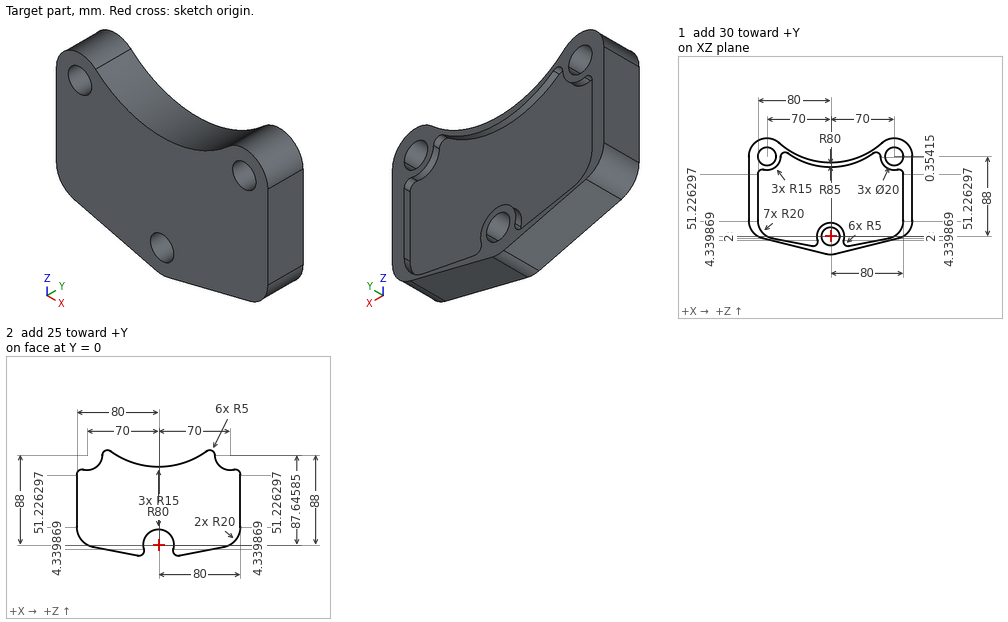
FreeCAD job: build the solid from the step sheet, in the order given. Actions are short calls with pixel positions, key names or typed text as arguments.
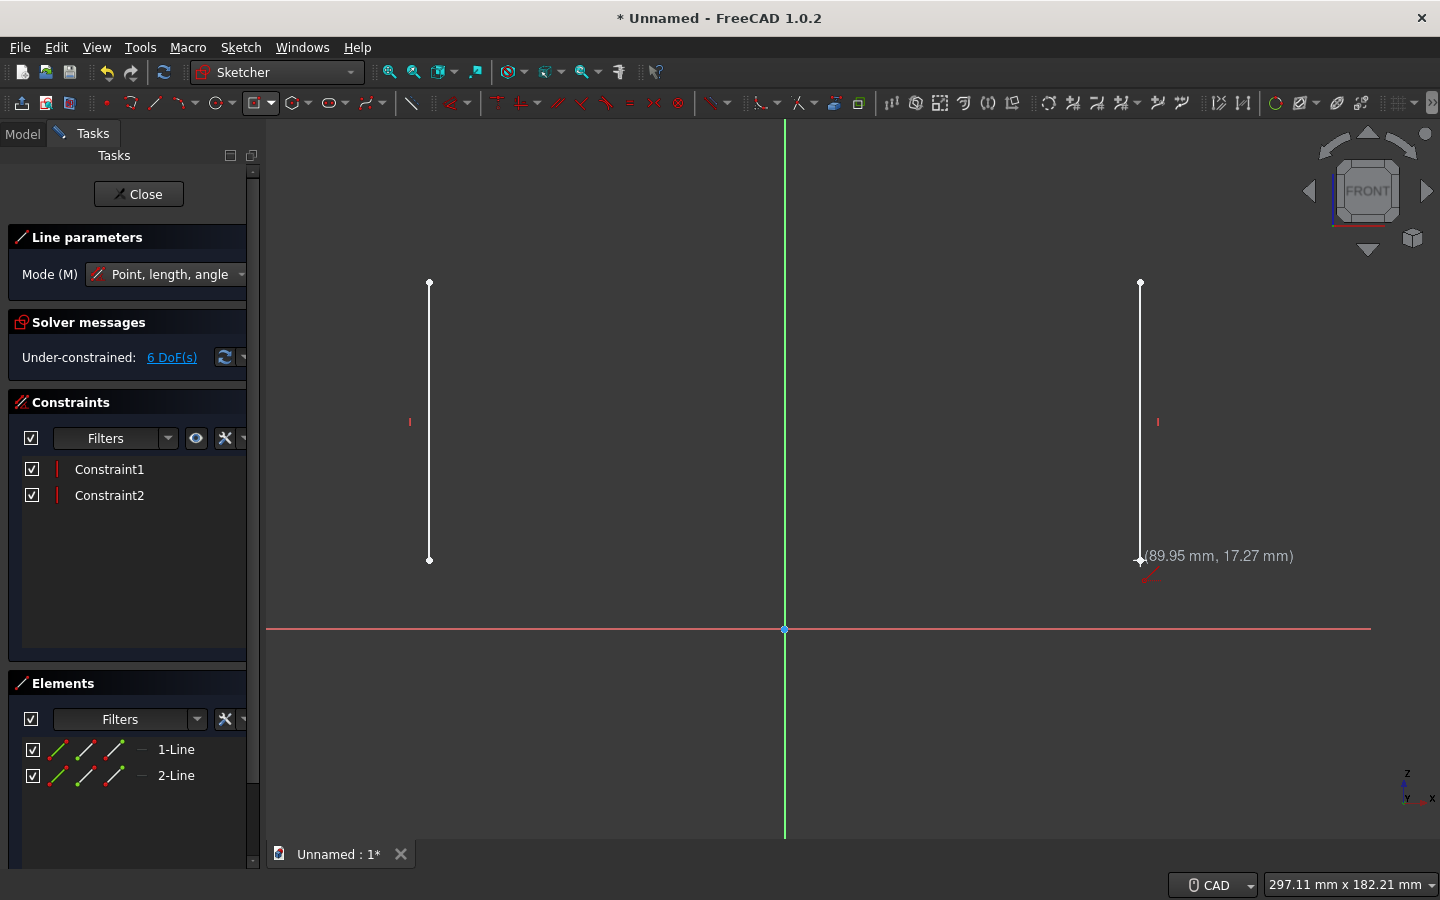
scroll(1080, 637, up, 4)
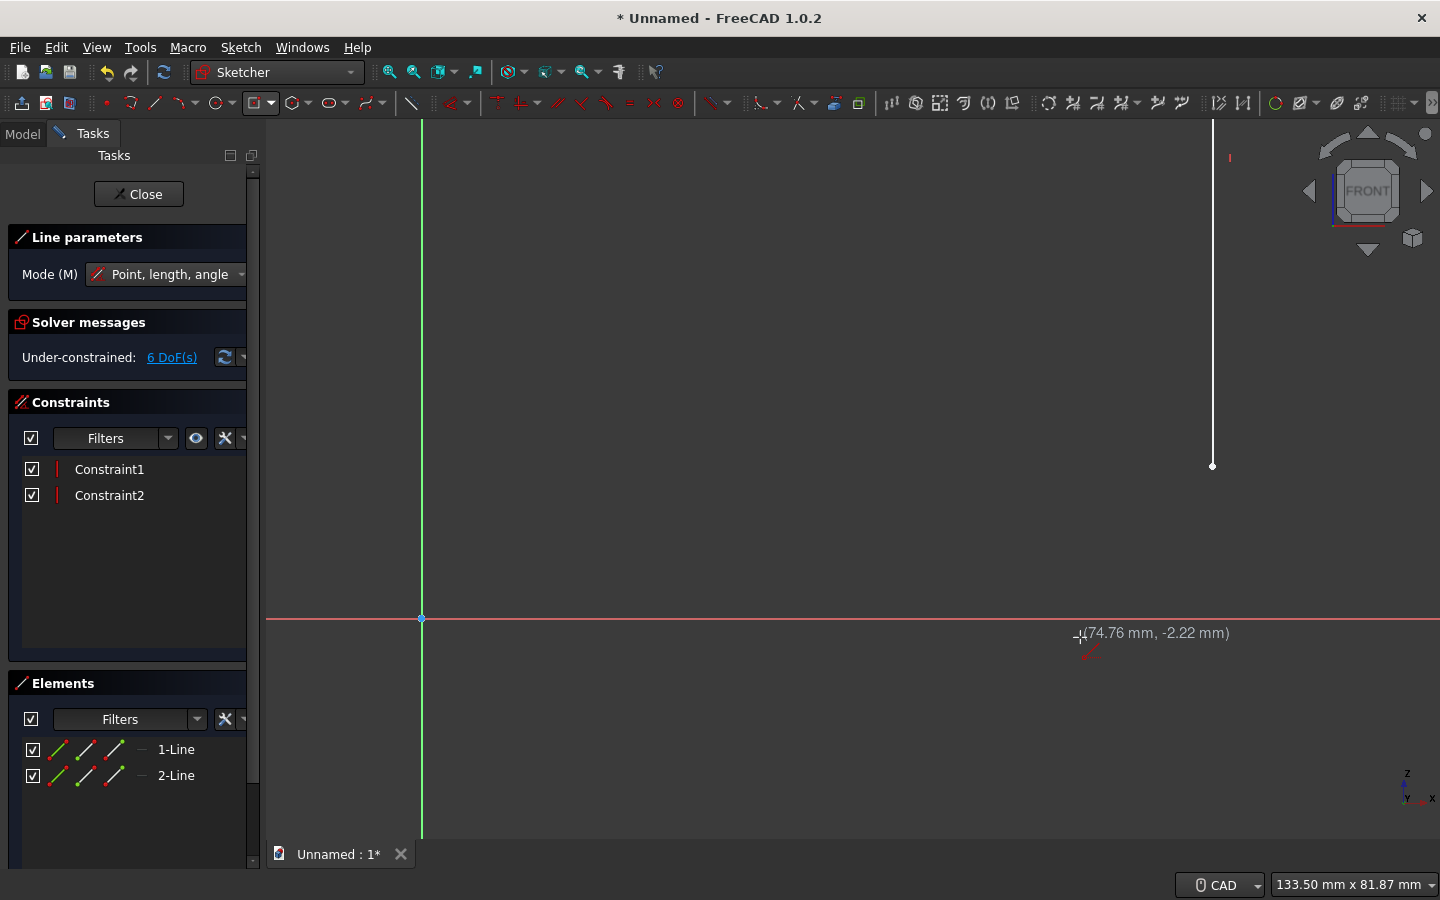
click(1080, 636)
click(464, 790)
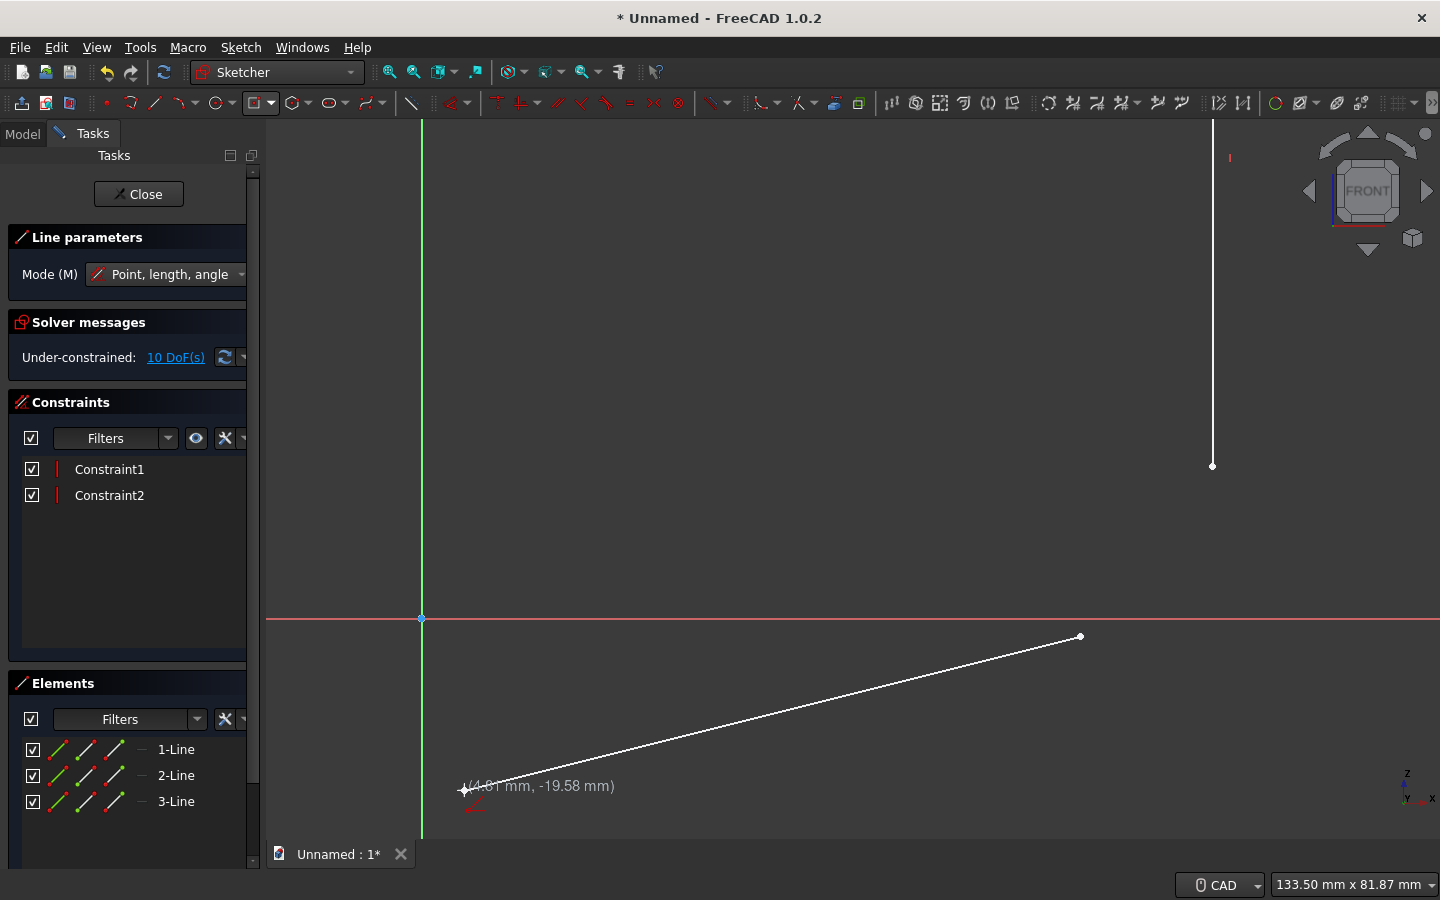
click(379, 790)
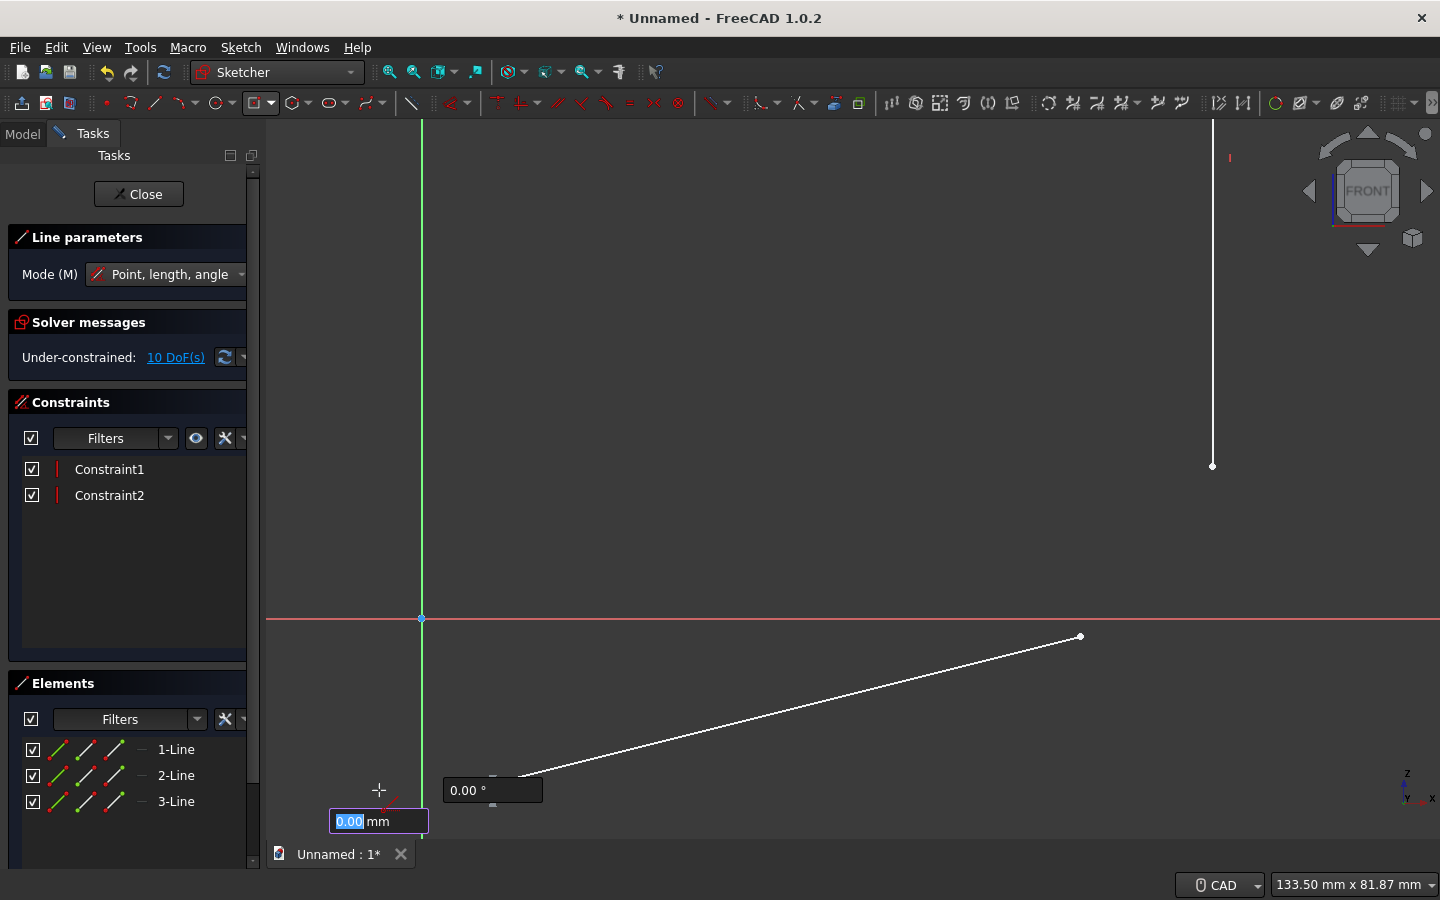
scroll(1081, 674, down, 4)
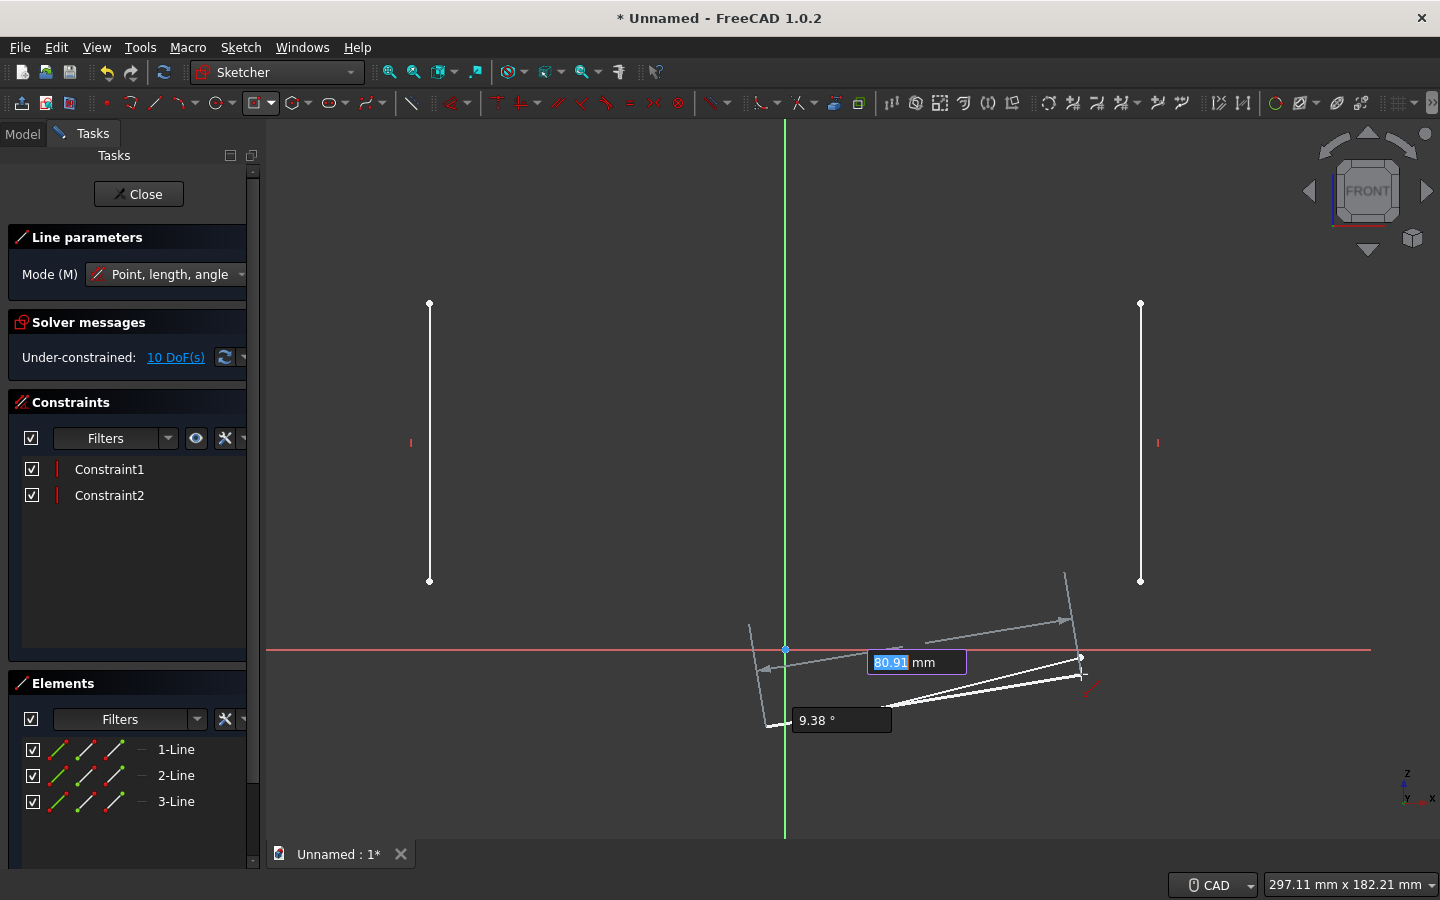
scroll(489, 658, up, 4)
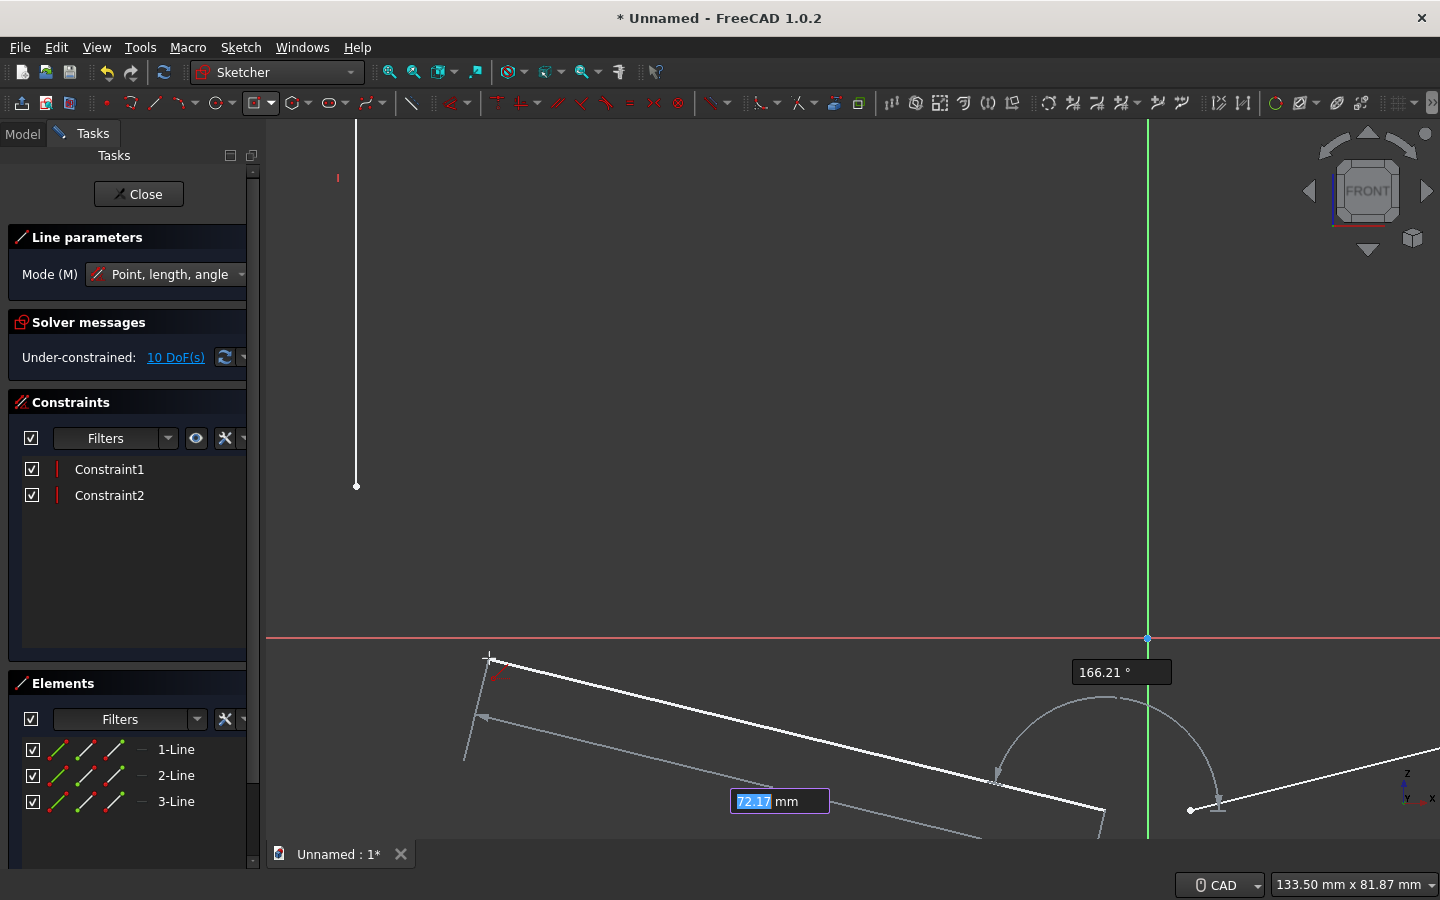
click(490, 656)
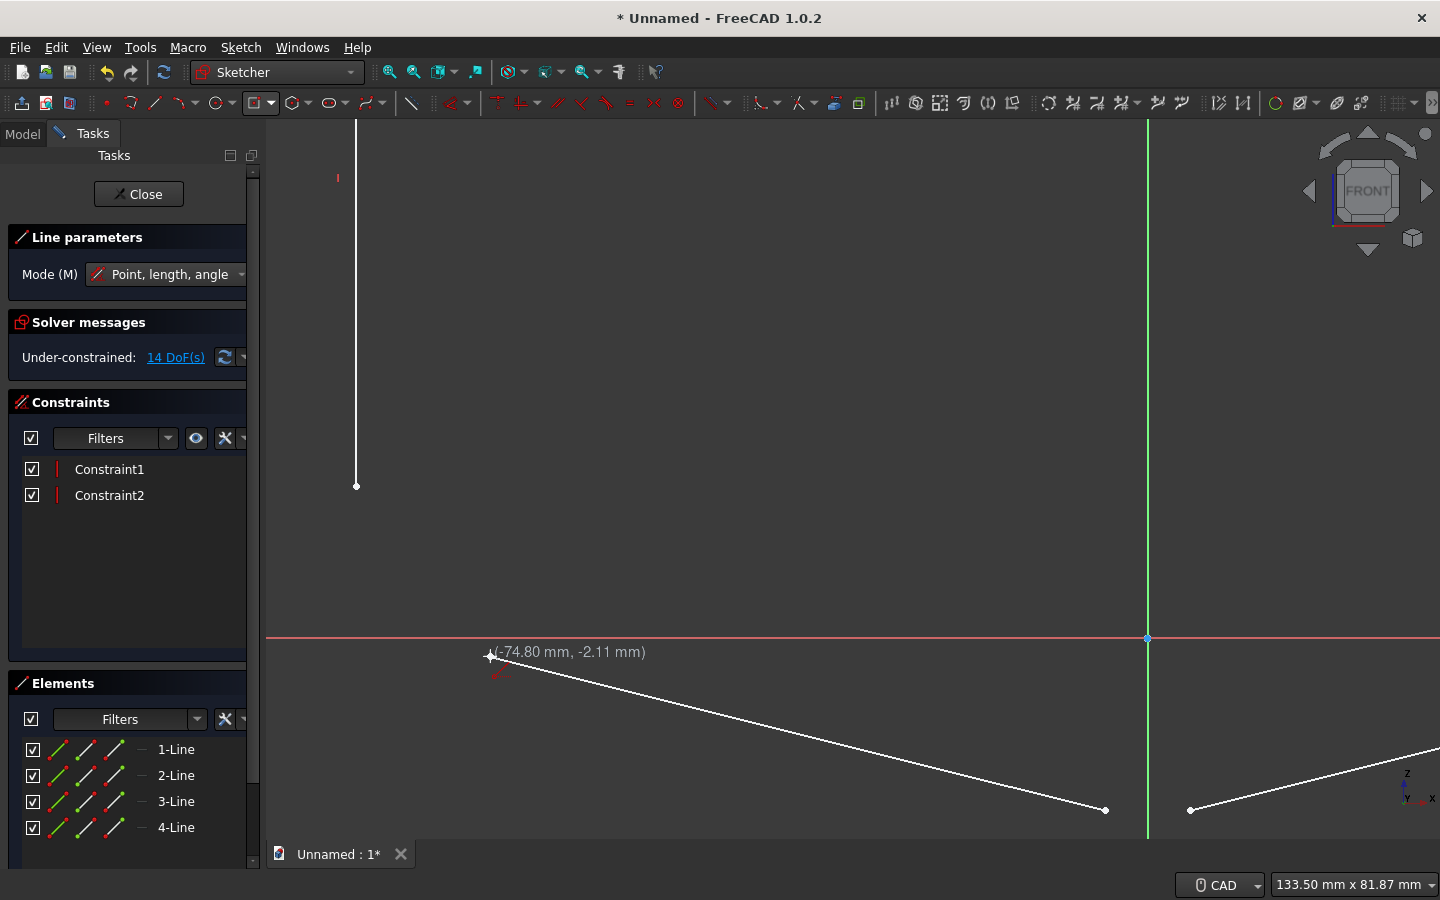
click(180, 104)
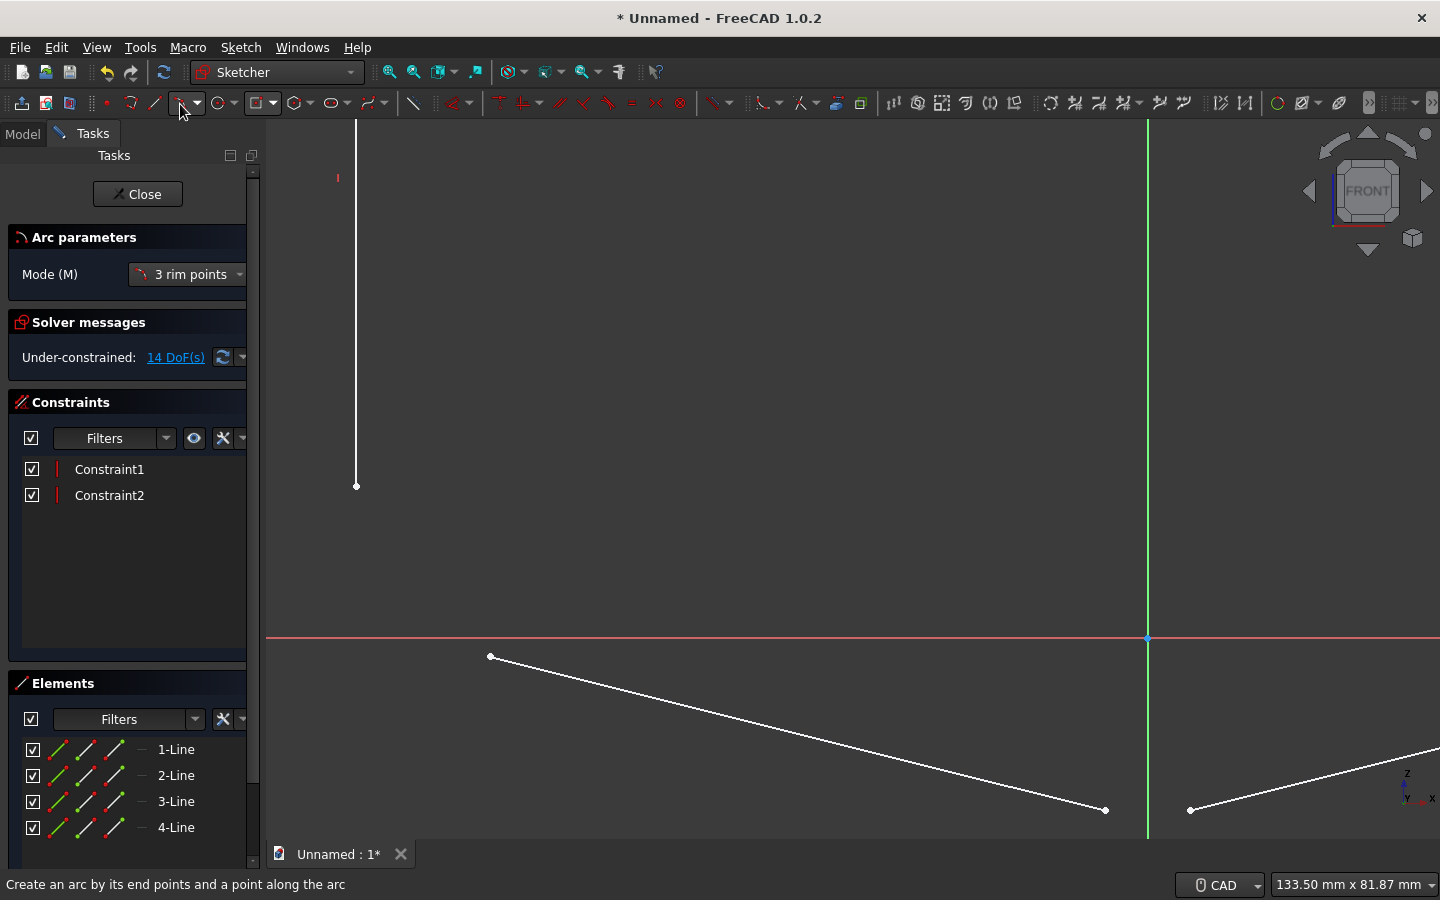
scroll(488, 658, down, 4)